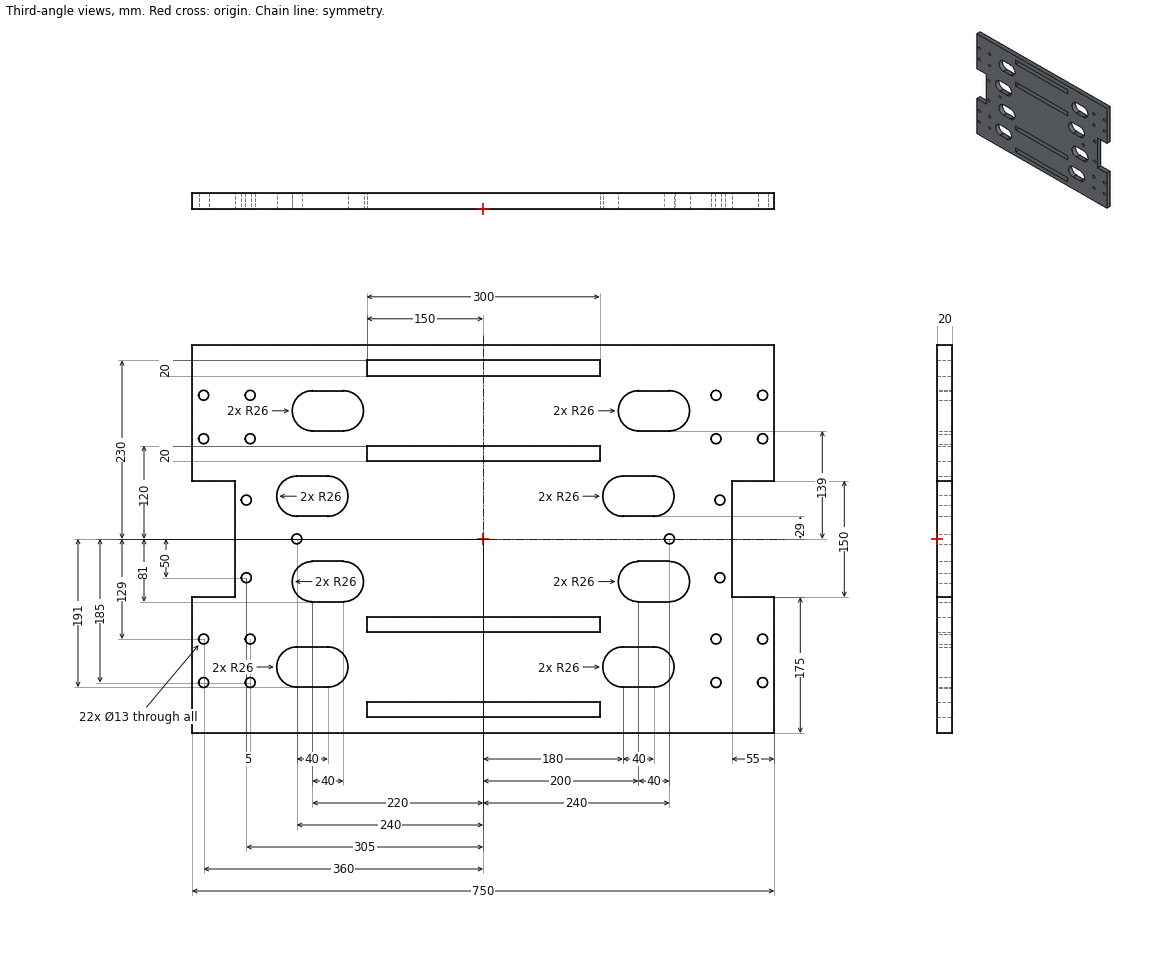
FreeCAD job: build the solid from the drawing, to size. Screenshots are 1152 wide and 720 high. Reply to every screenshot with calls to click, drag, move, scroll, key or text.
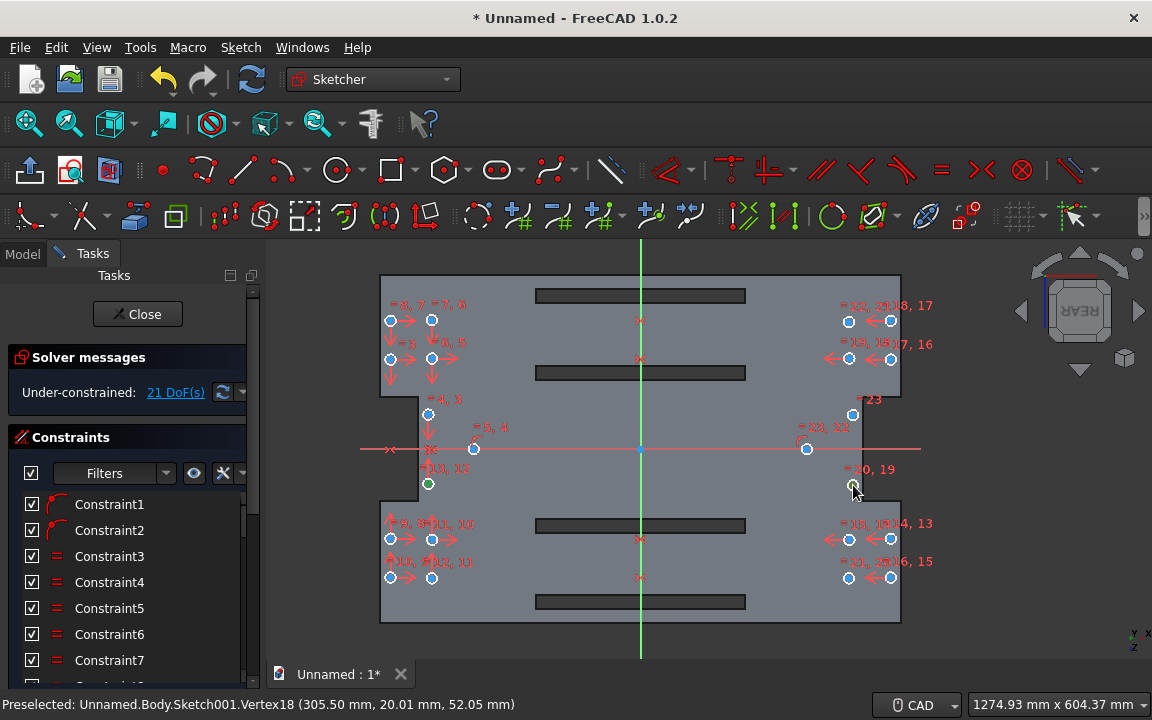
click(641, 605)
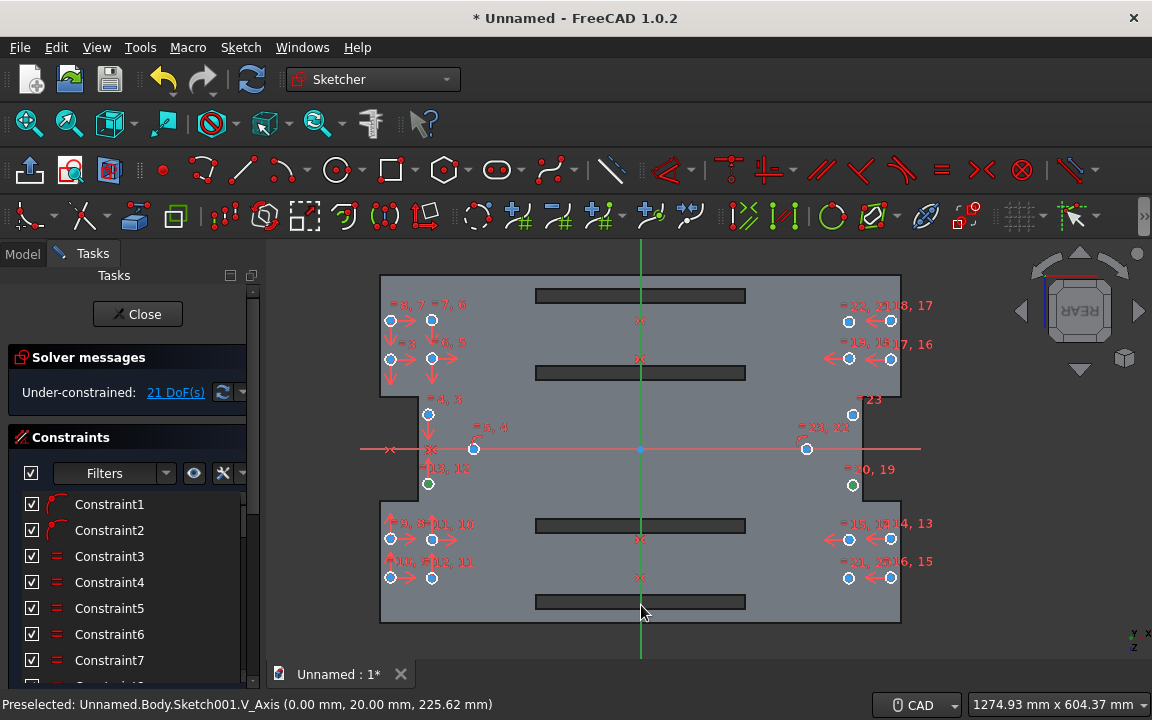
click(982, 170)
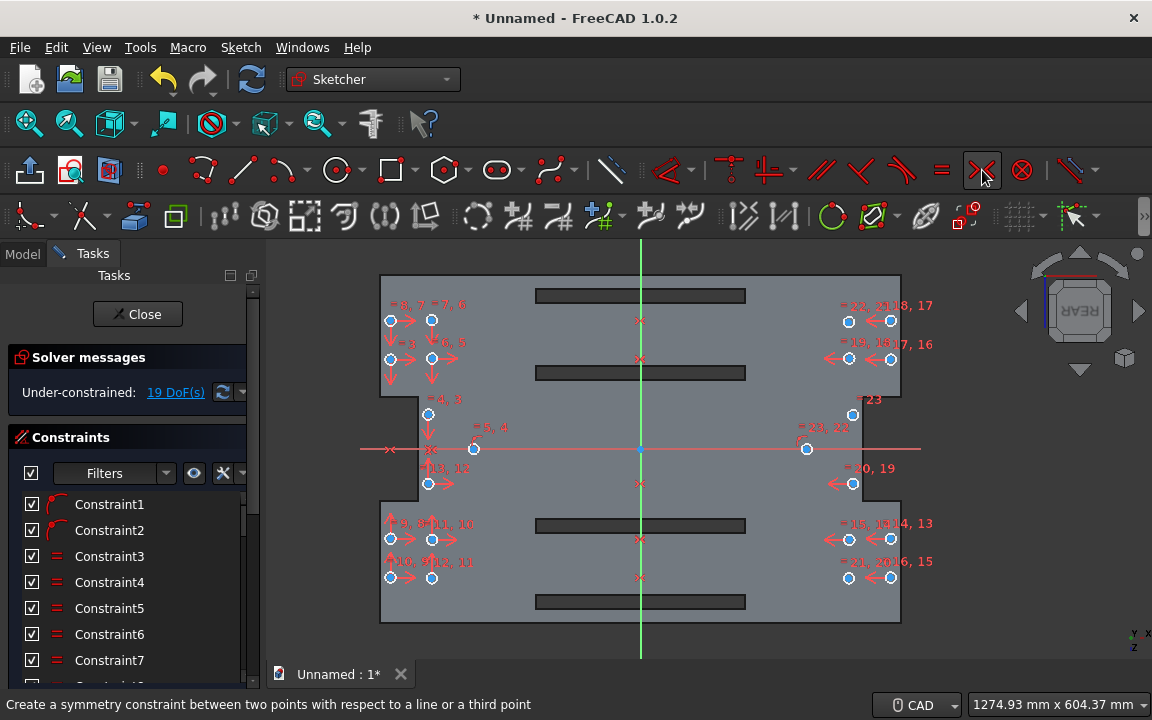
click(432, 578)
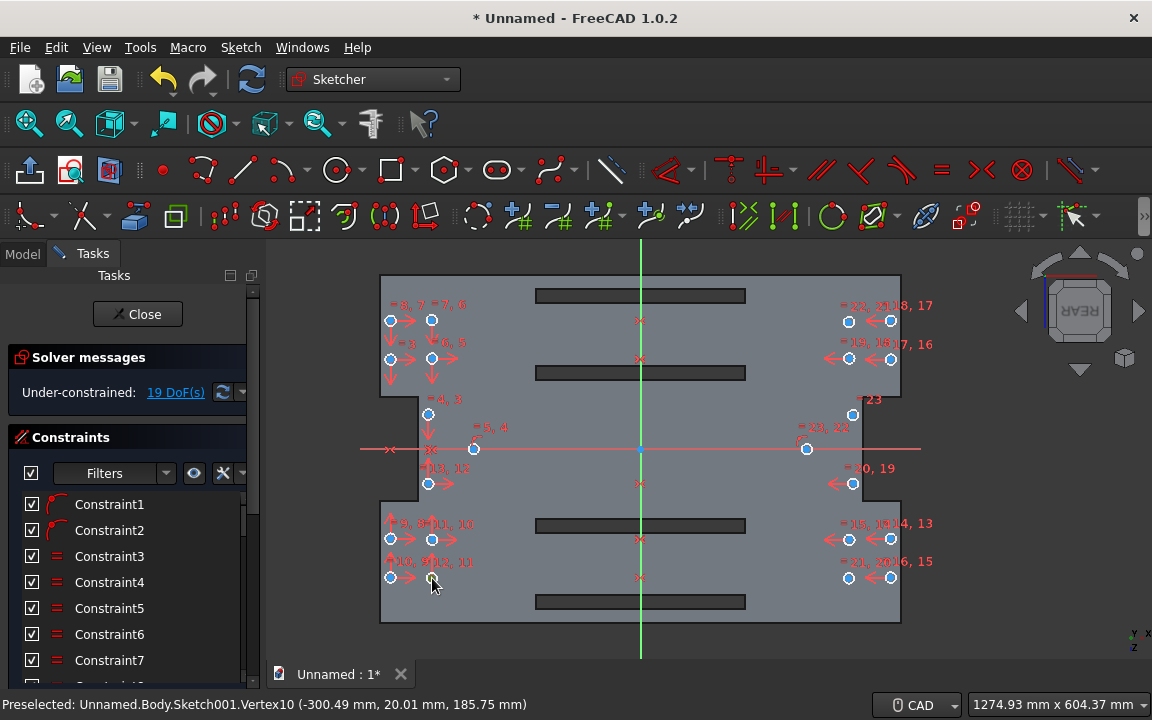
click(849, 578)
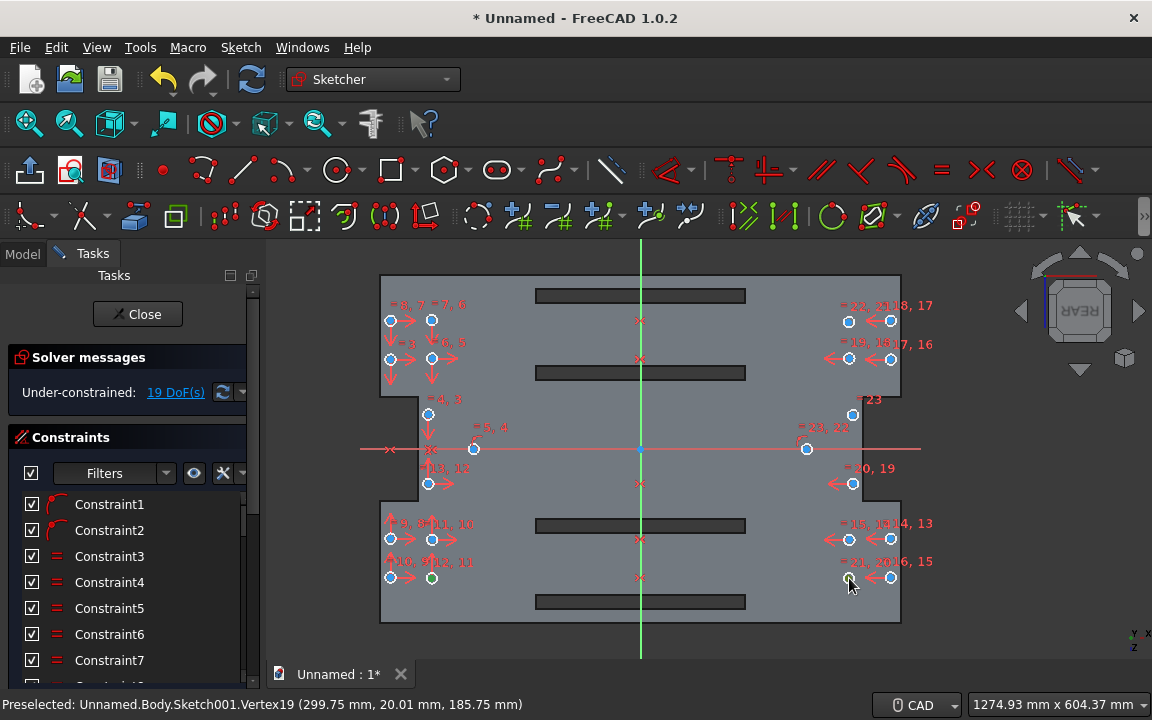
click(641, 605)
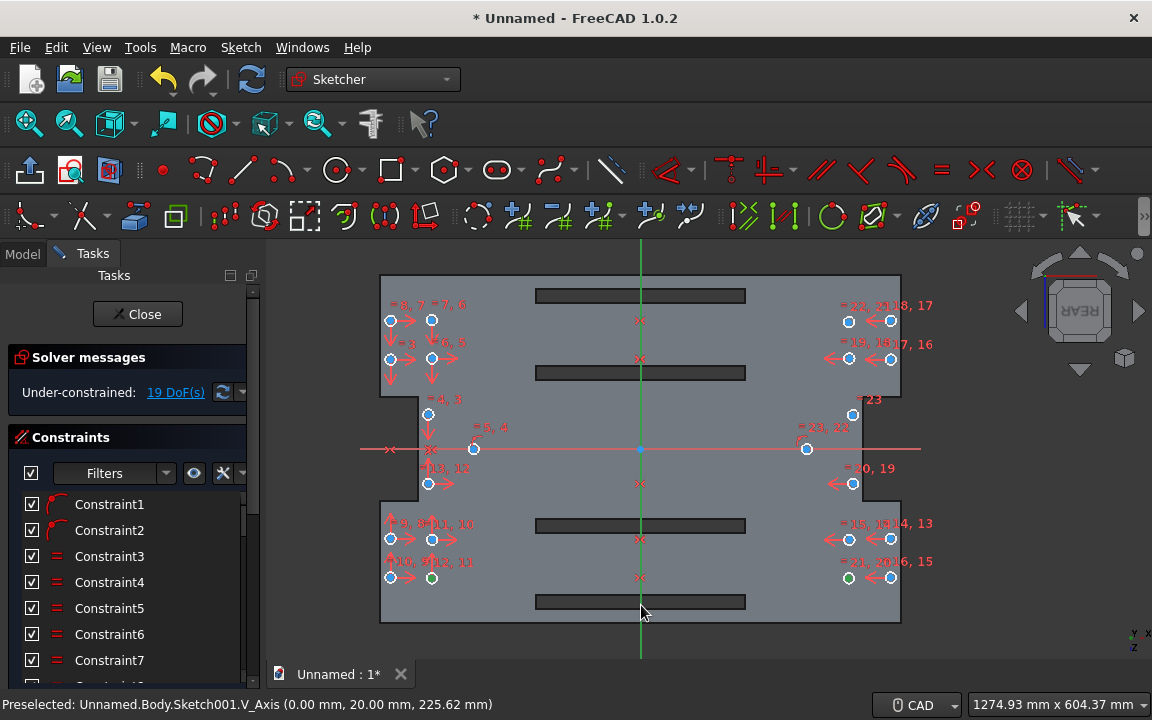
click(982, 170)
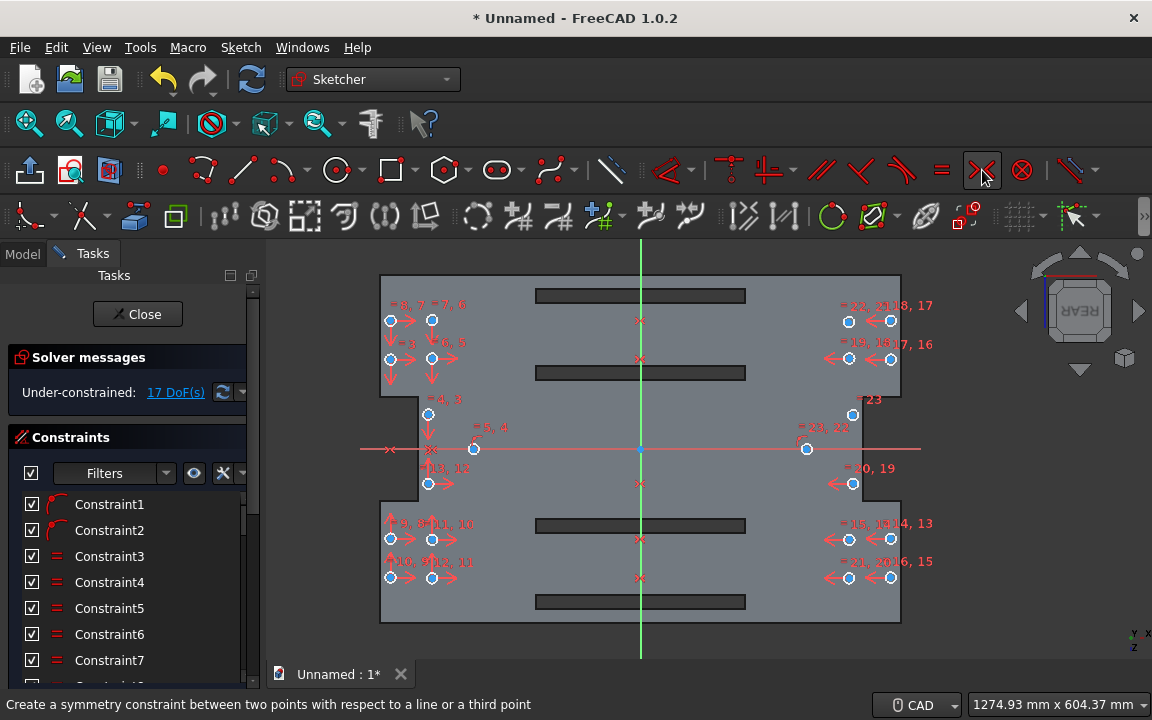
click(432, 320)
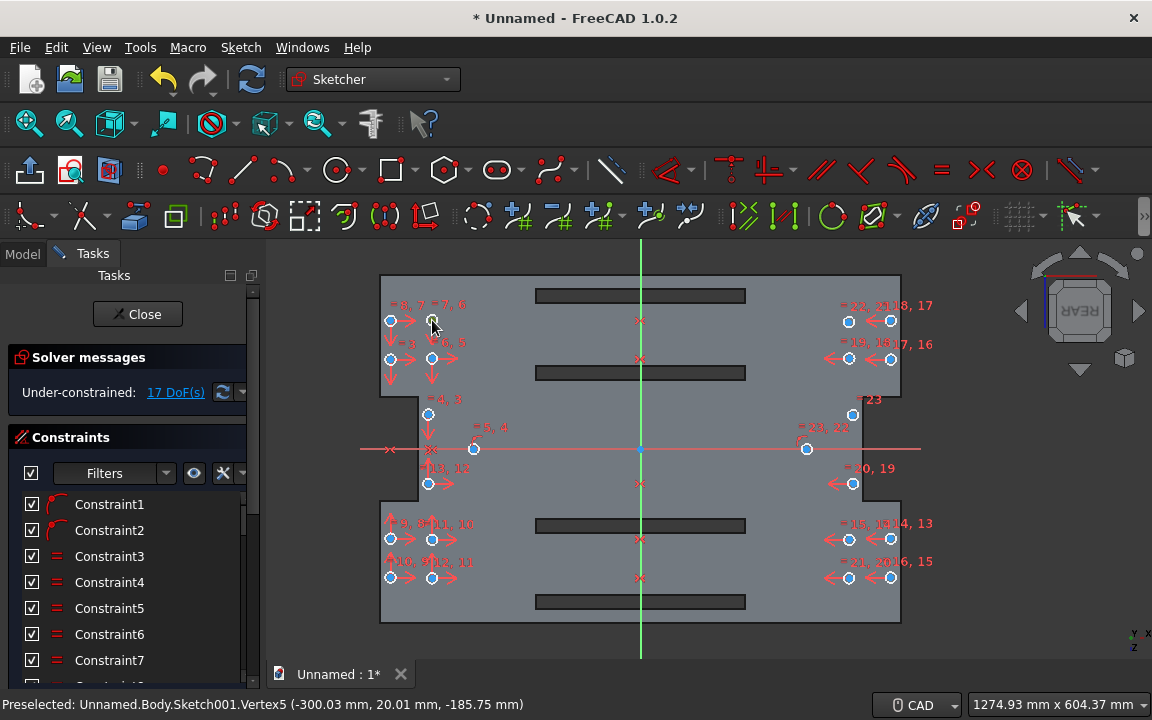
click(849, 322)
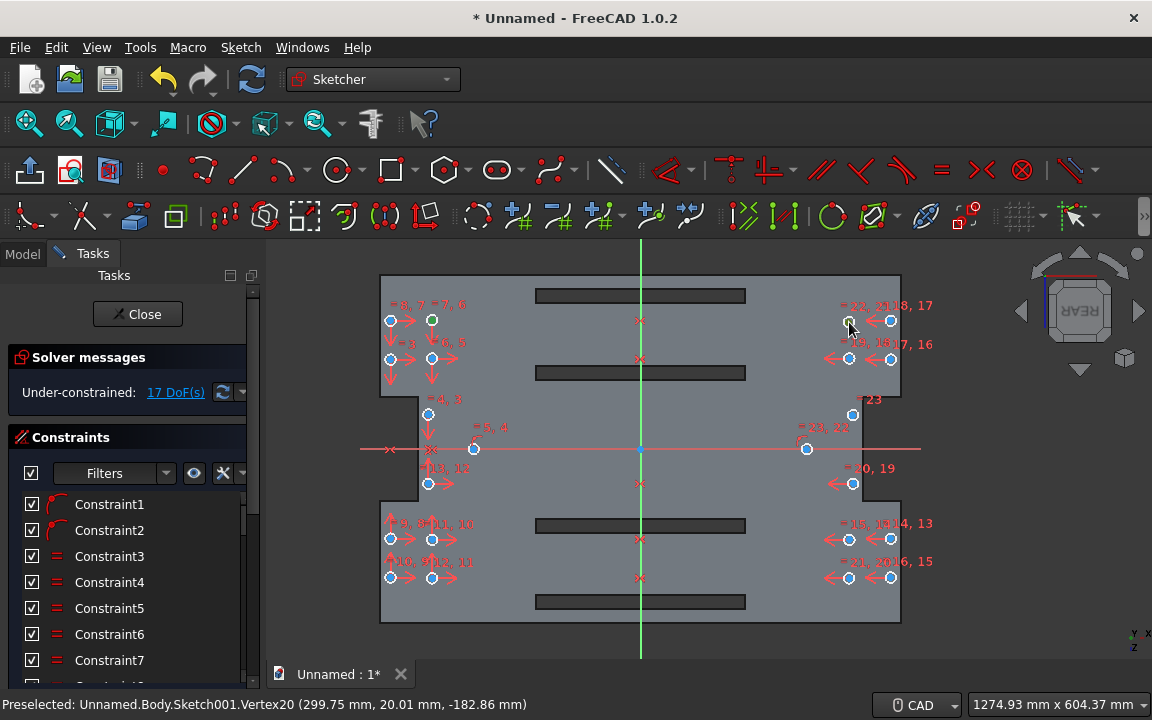
click(641, 605)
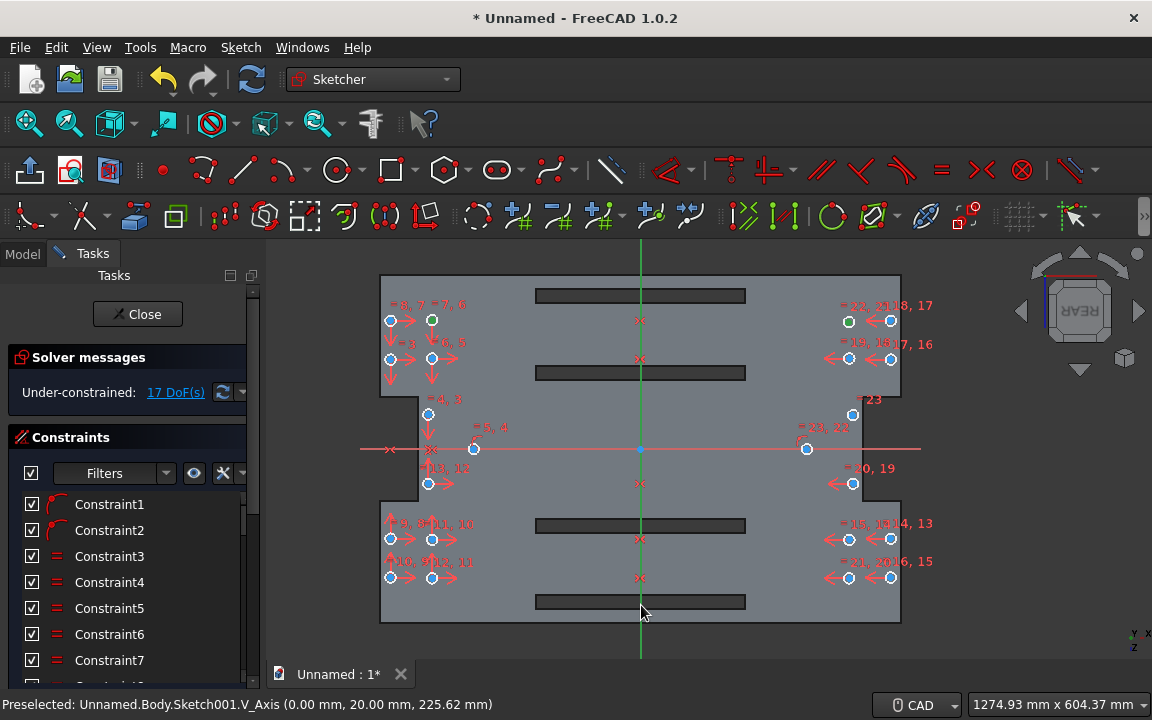
click(982, 170)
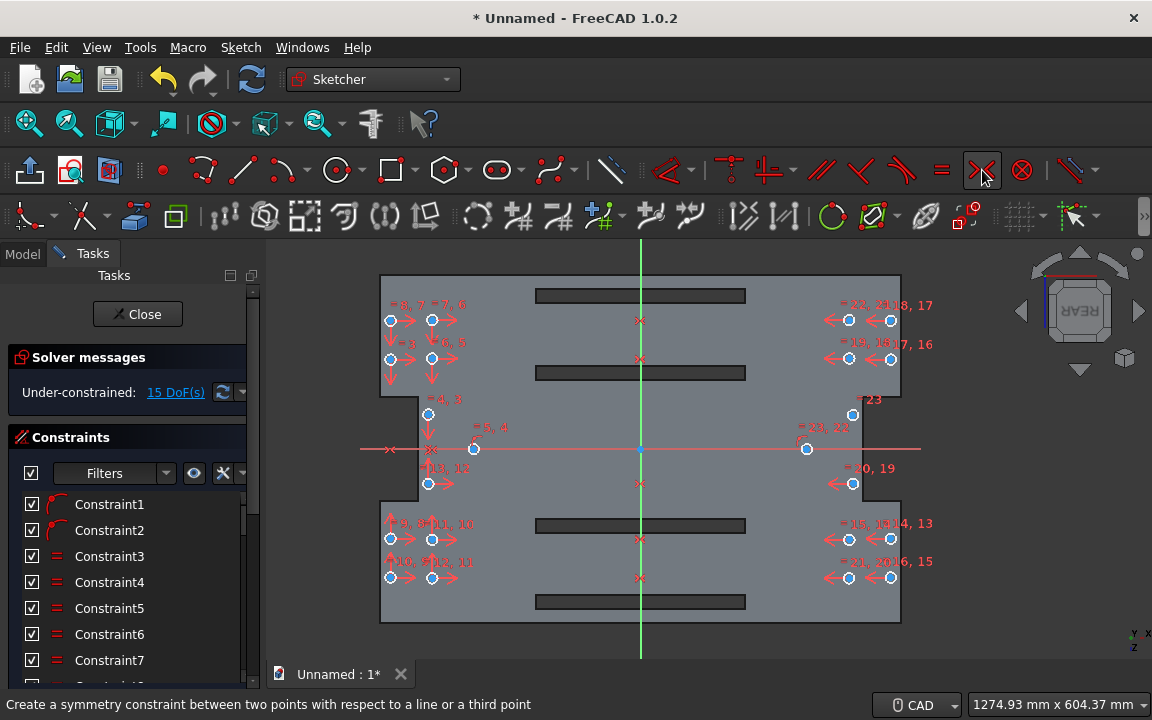
click(428, 415)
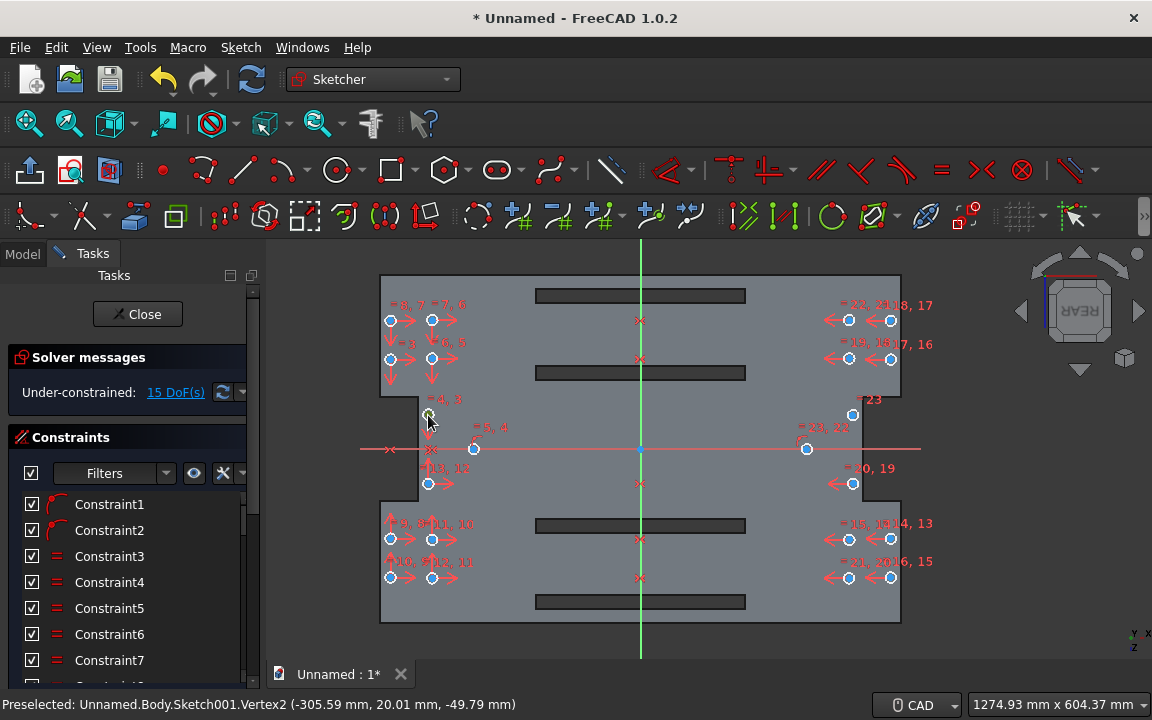
click(853, 415)